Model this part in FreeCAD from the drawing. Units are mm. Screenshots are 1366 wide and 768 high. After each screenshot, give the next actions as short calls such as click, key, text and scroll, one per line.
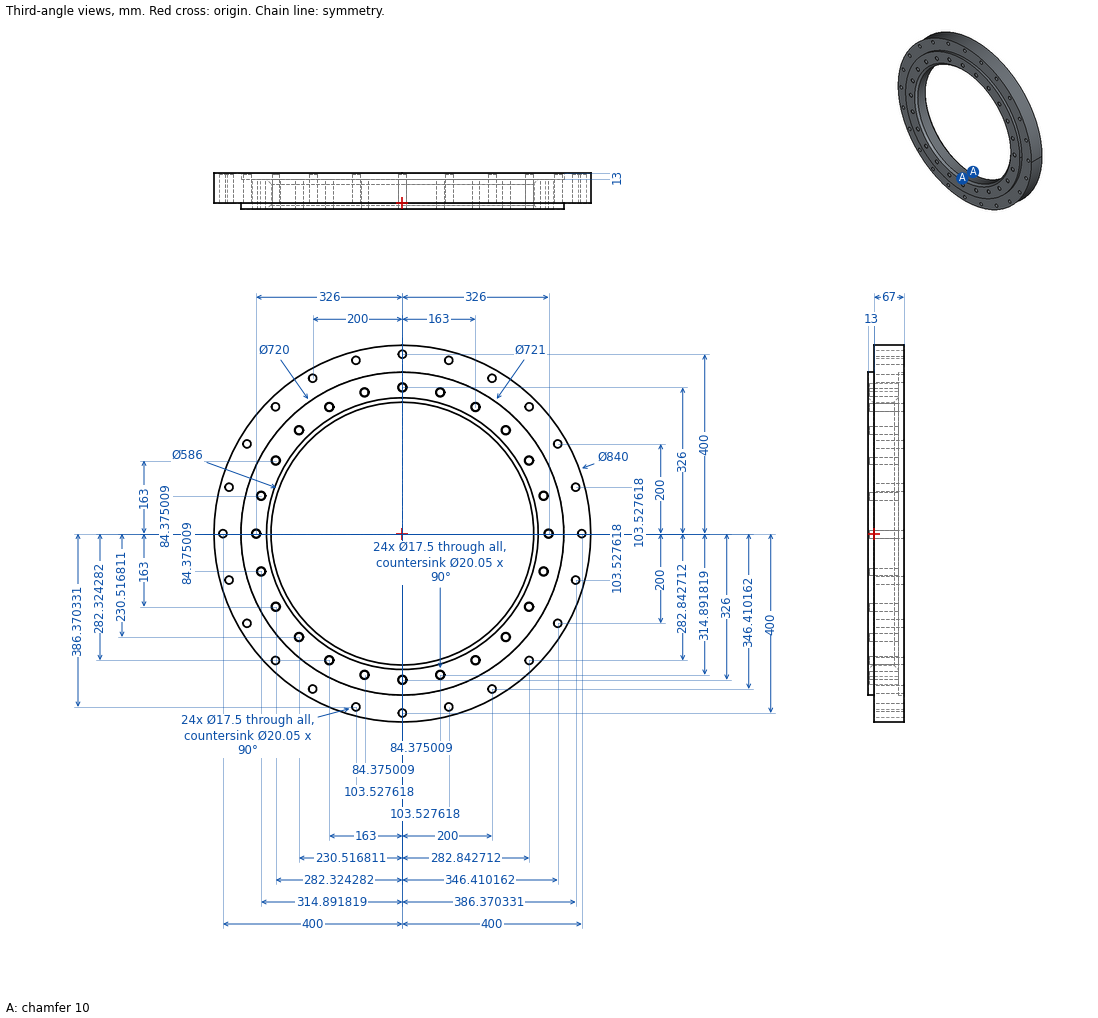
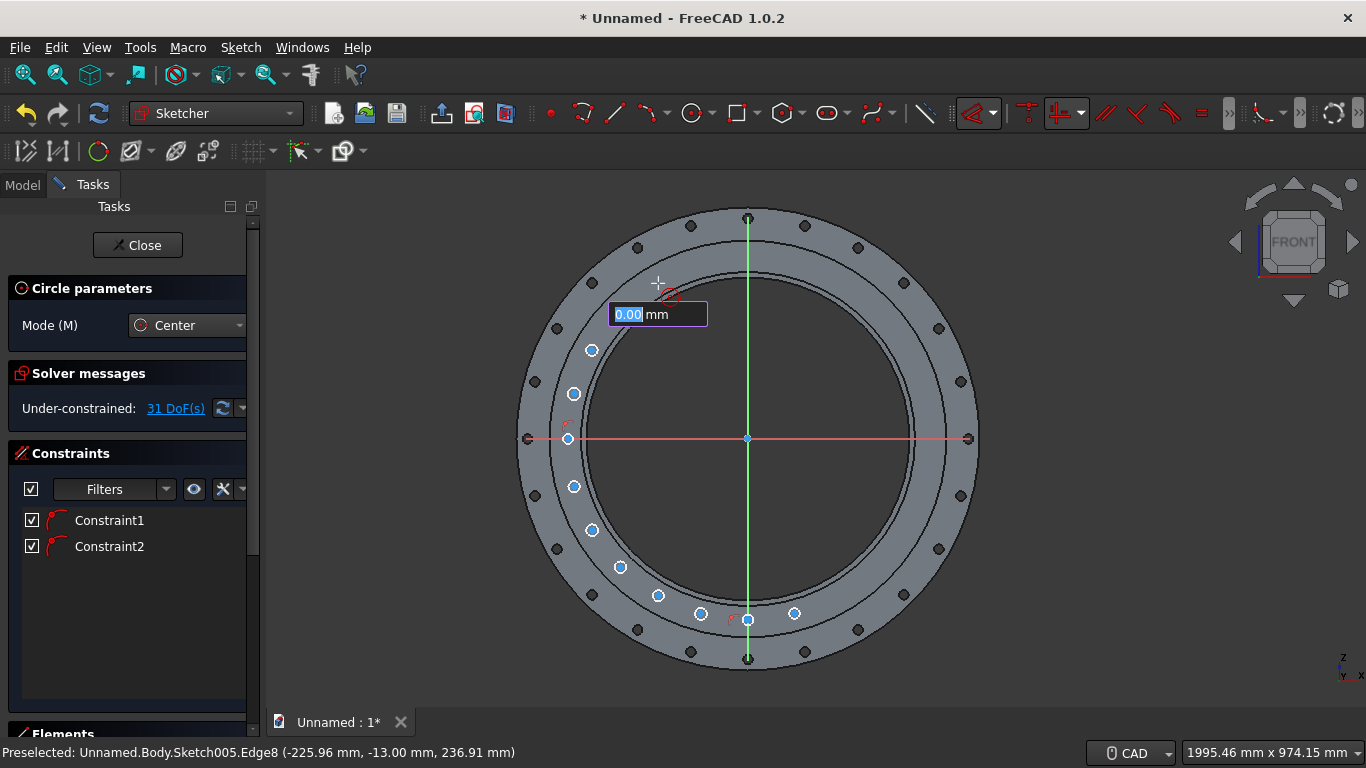
scroll(662, 280, up, 6)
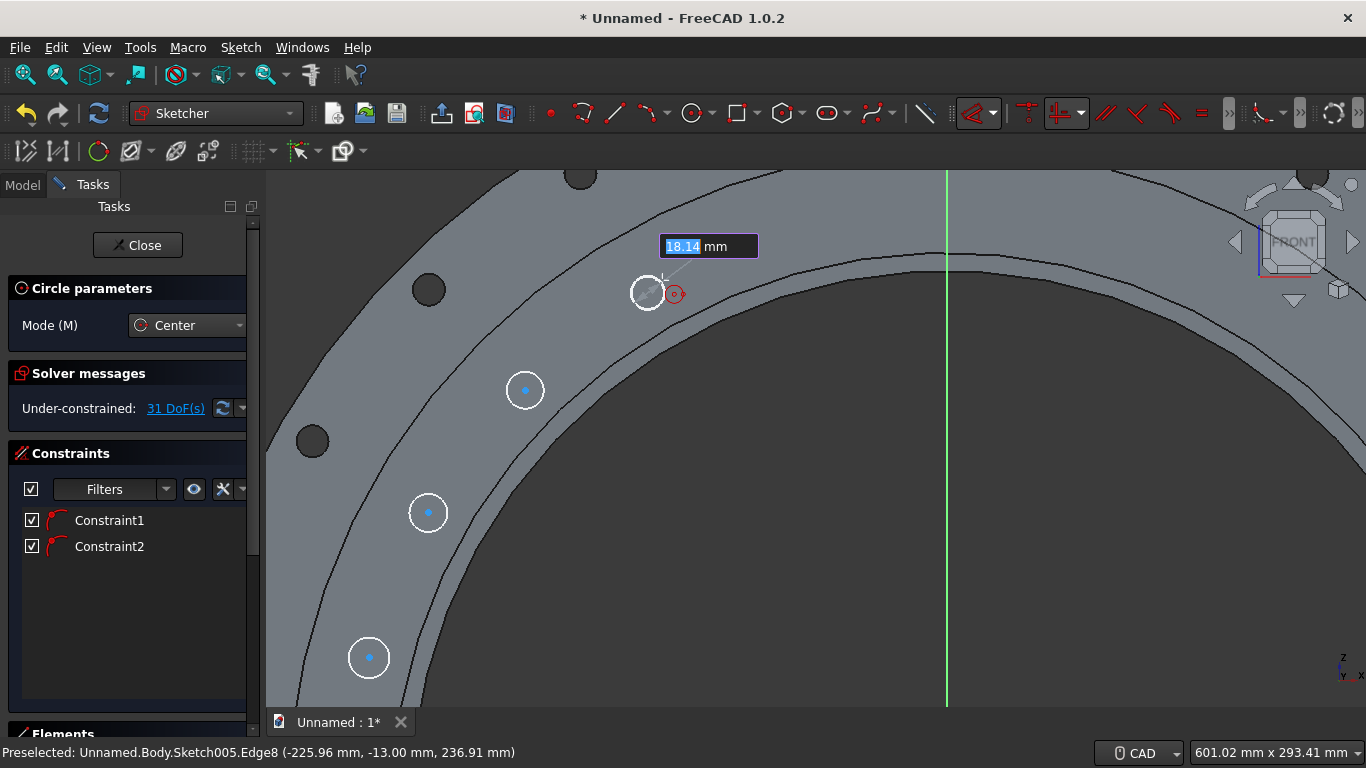
click(660, 279)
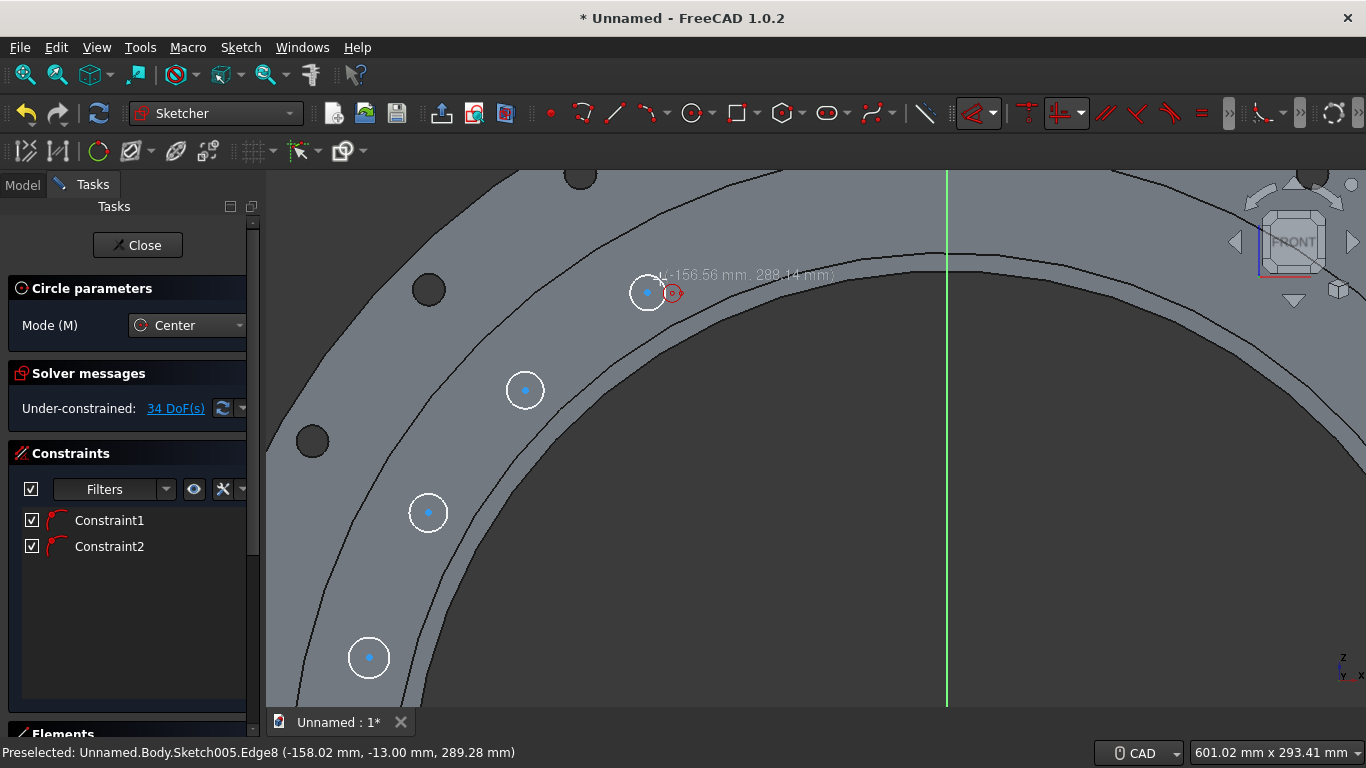
scroll(792, 231, up, 2)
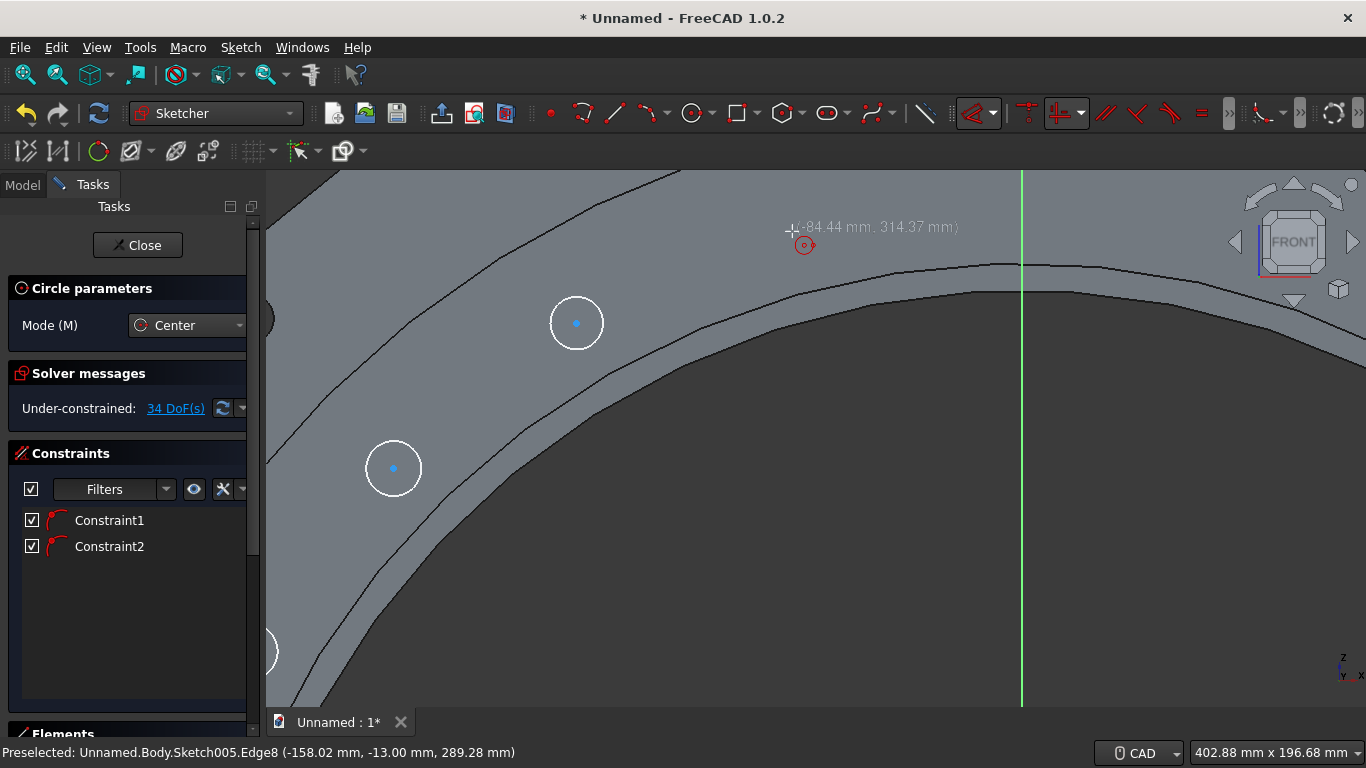
scroll(678, 273, down, 8)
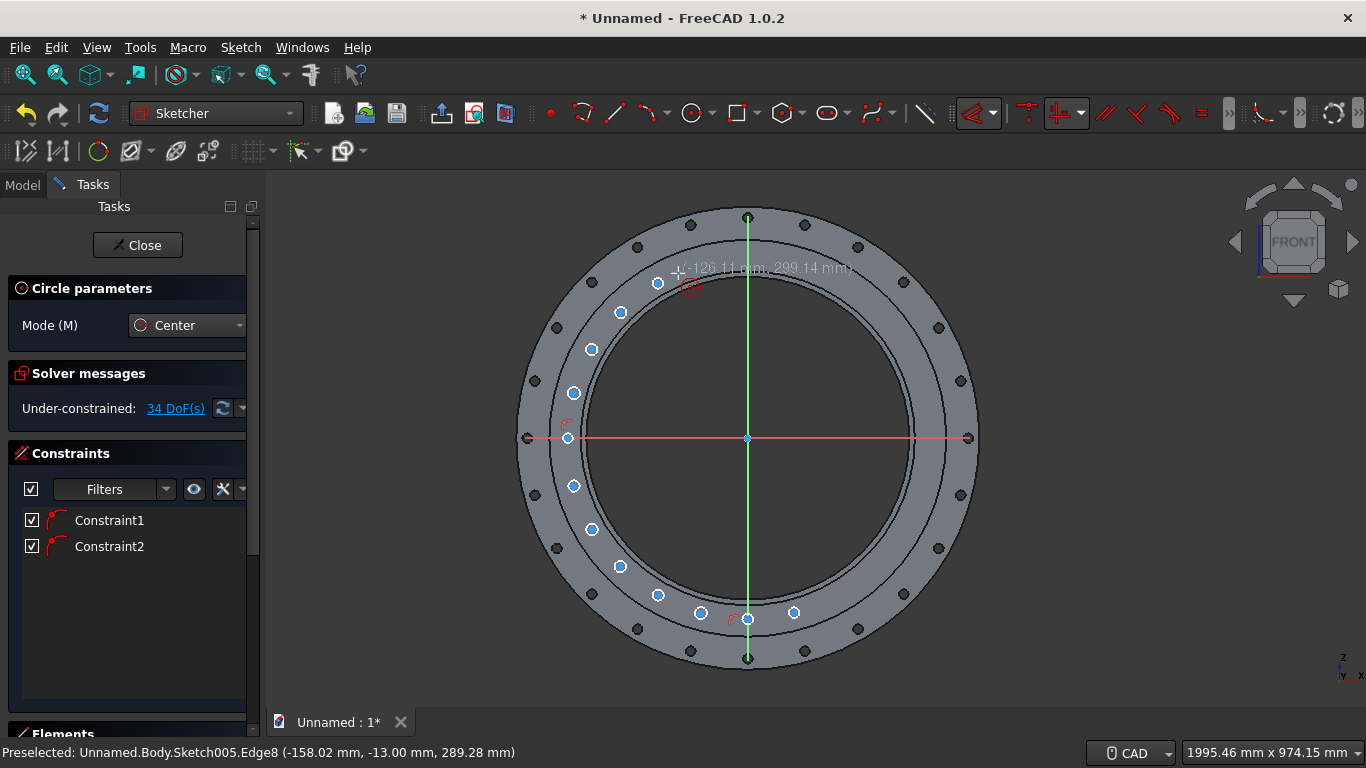
click(701, 265)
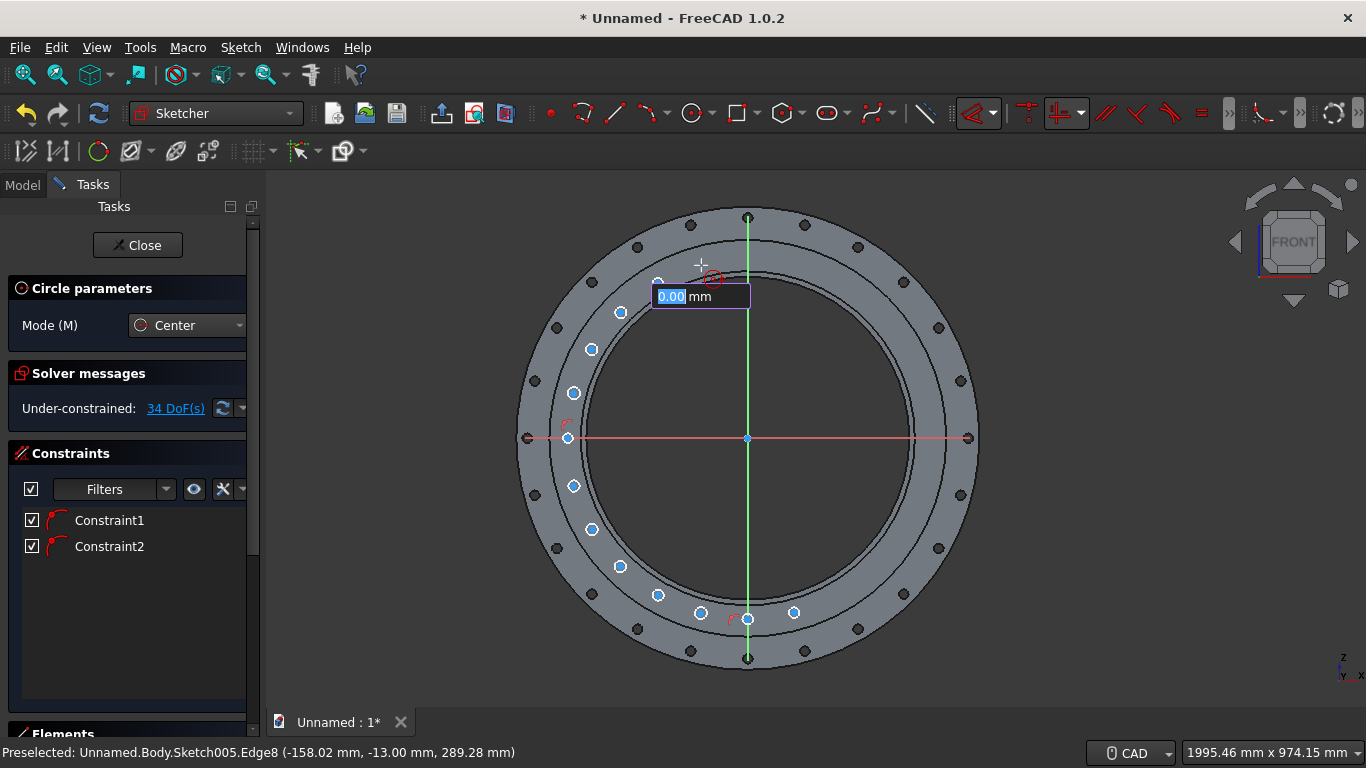
scroll(705, 261, up, 6)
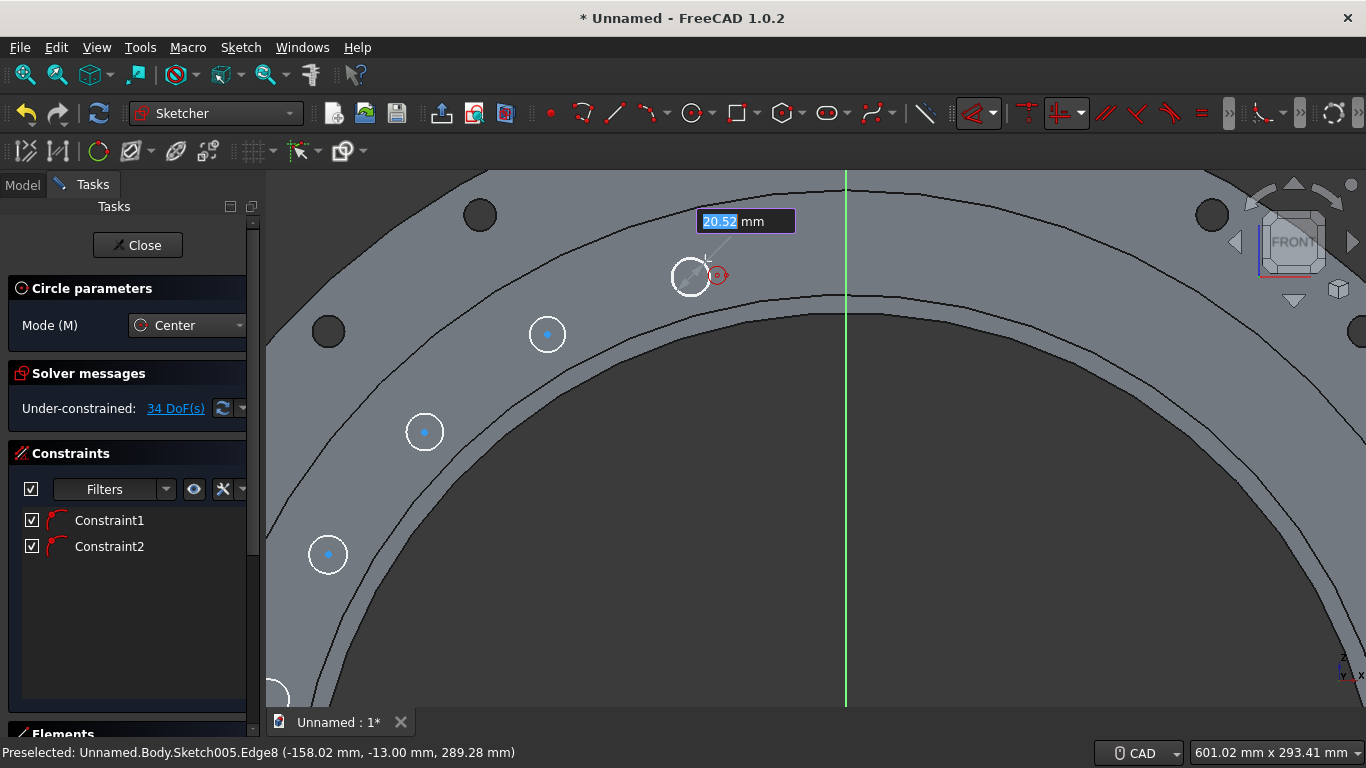
click(703, 261)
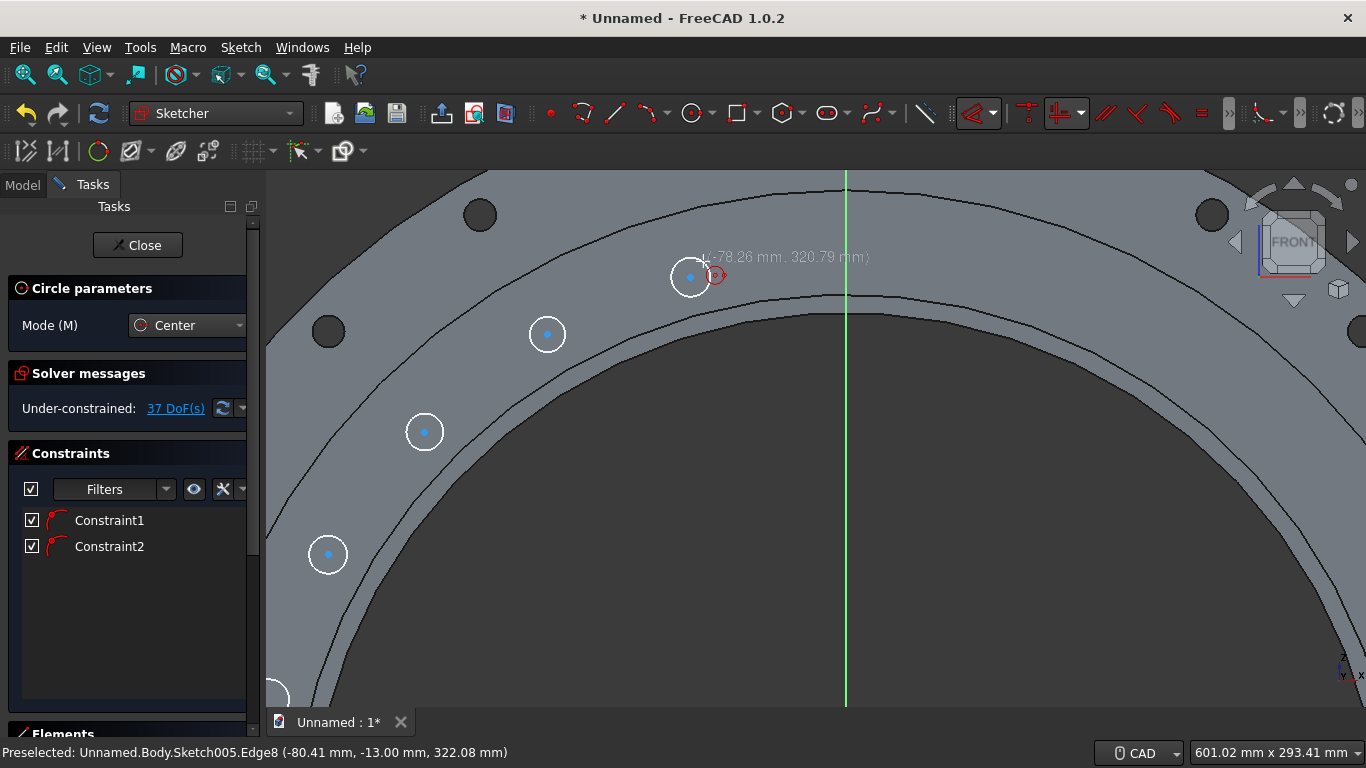
scroll(846, 252, up, 2)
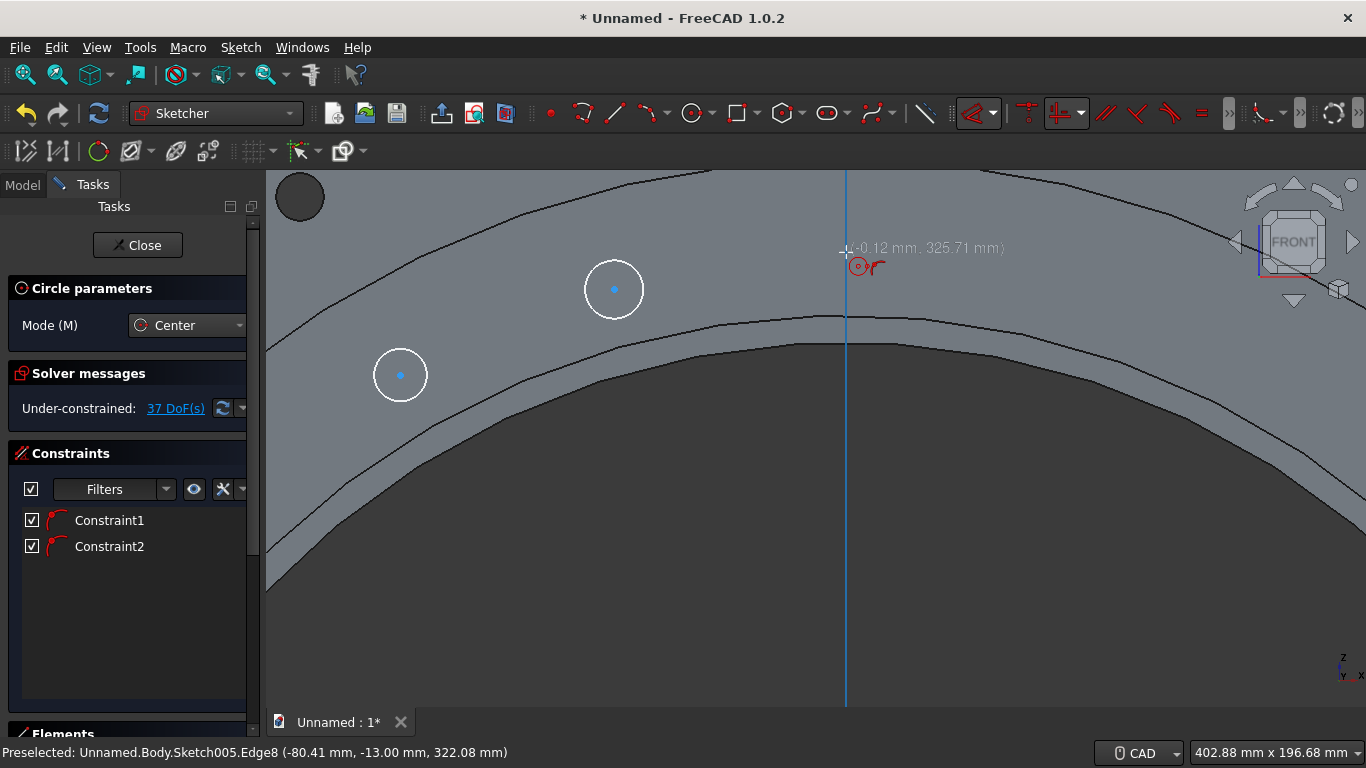
scroll(723, 260, down, 8)